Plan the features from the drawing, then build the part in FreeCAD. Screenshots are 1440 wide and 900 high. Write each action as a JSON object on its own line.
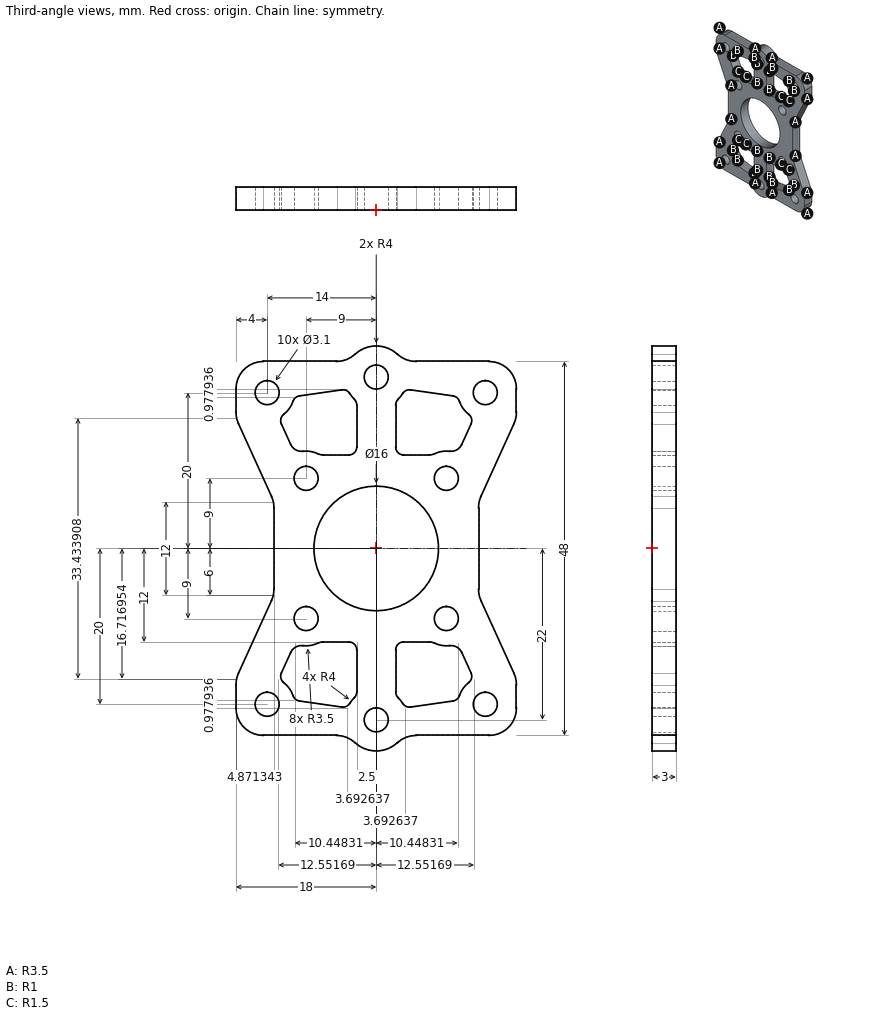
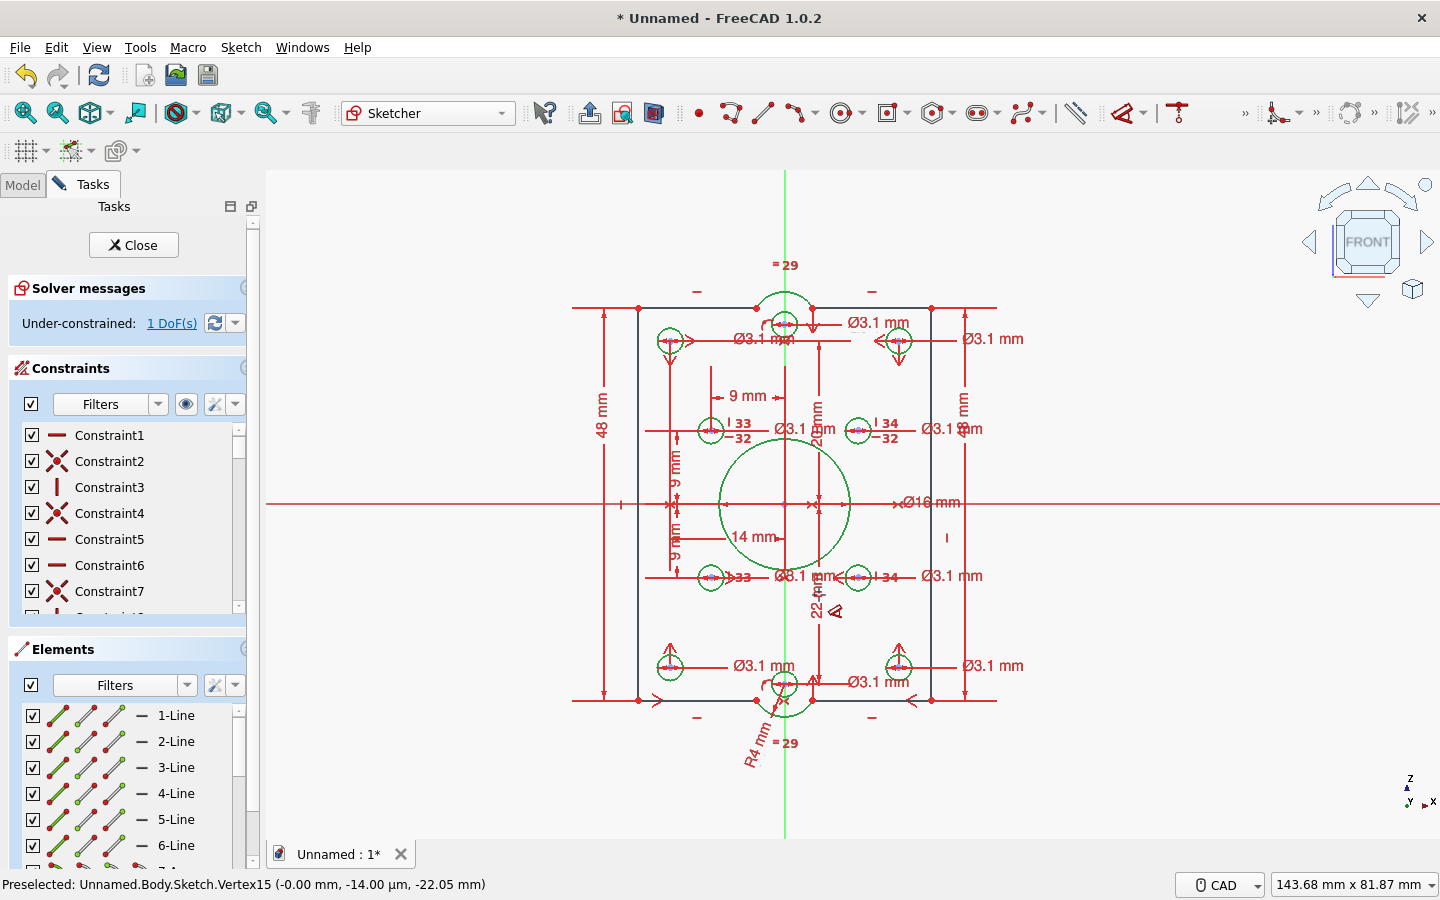
{"action": "left_click", "coordinate": [638, 308]}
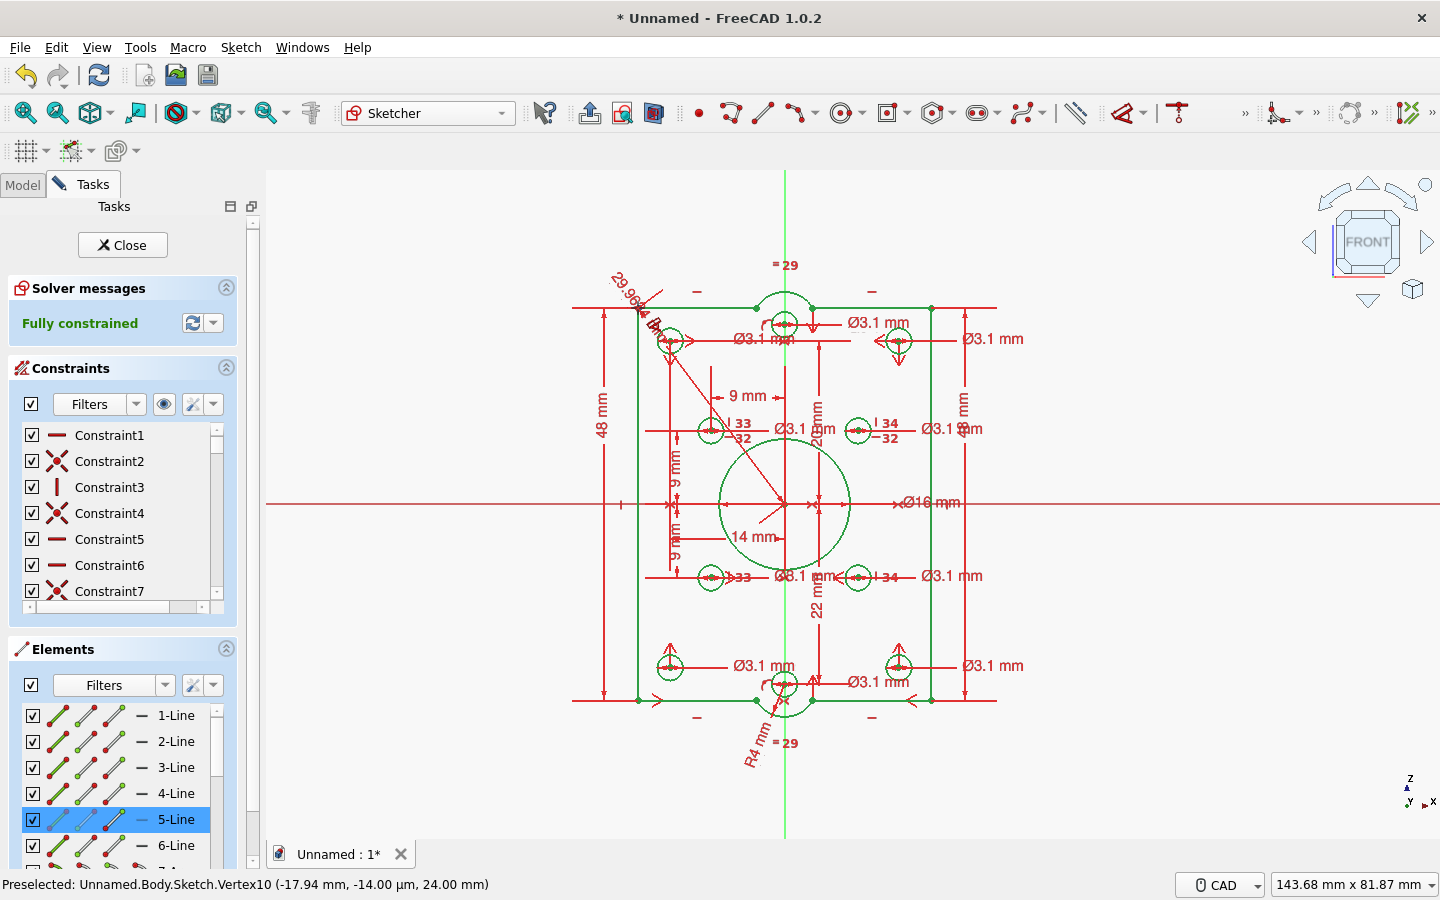
{"action": "left_click", "coordinate": [670, 341]}
{"action": "left_click", "coordinate": [654, 274]}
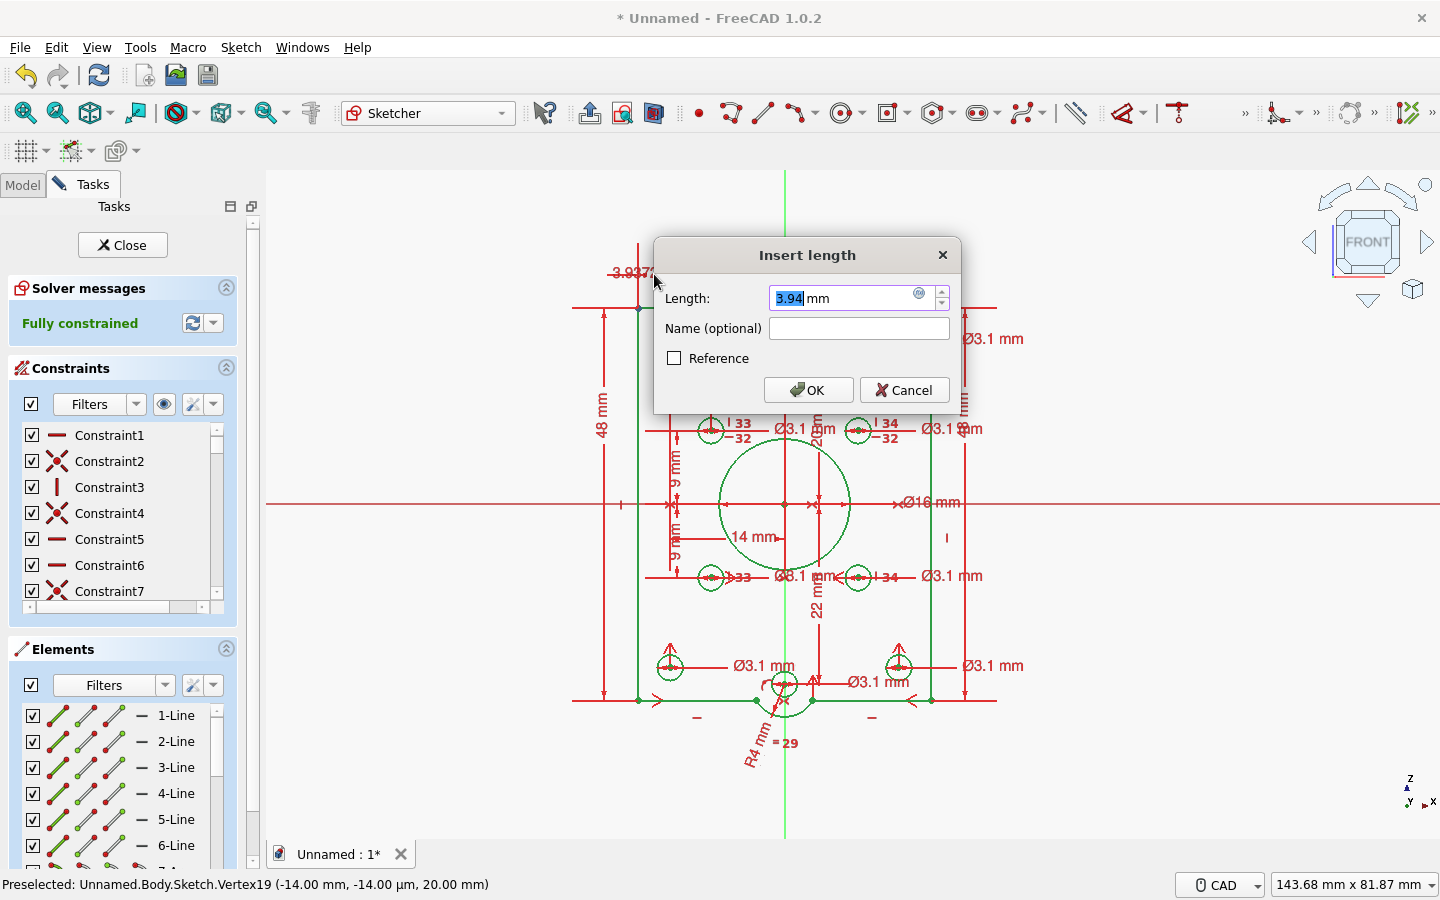
{"action": "type", "text": "4"}
{"action": "key", "text": "Return"}
{"action": "key", "text": "Escape"}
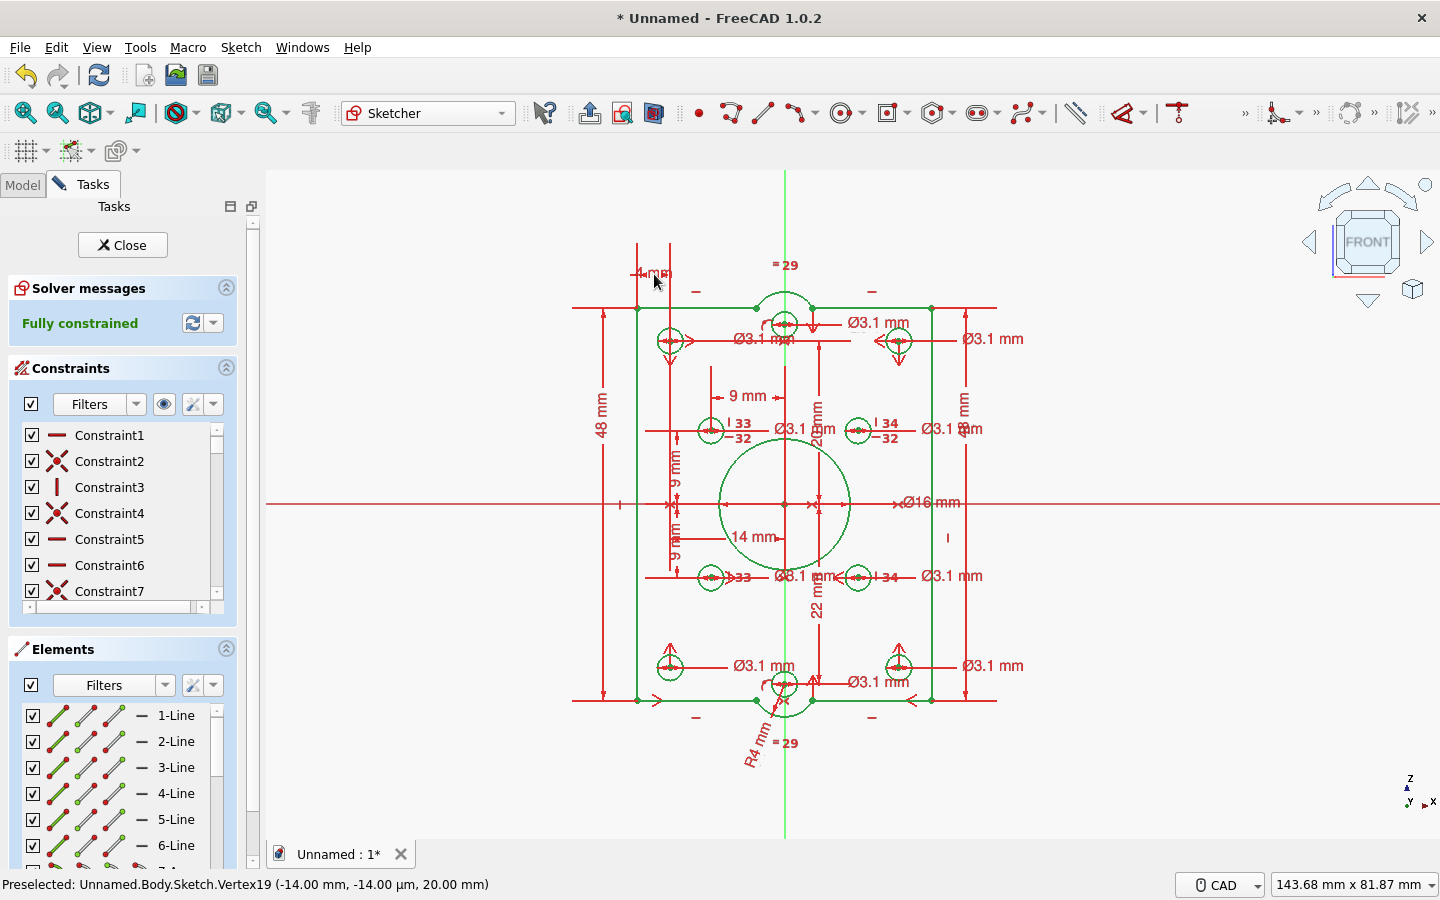
{"action": "left_click", "coordinate": [123, 245]}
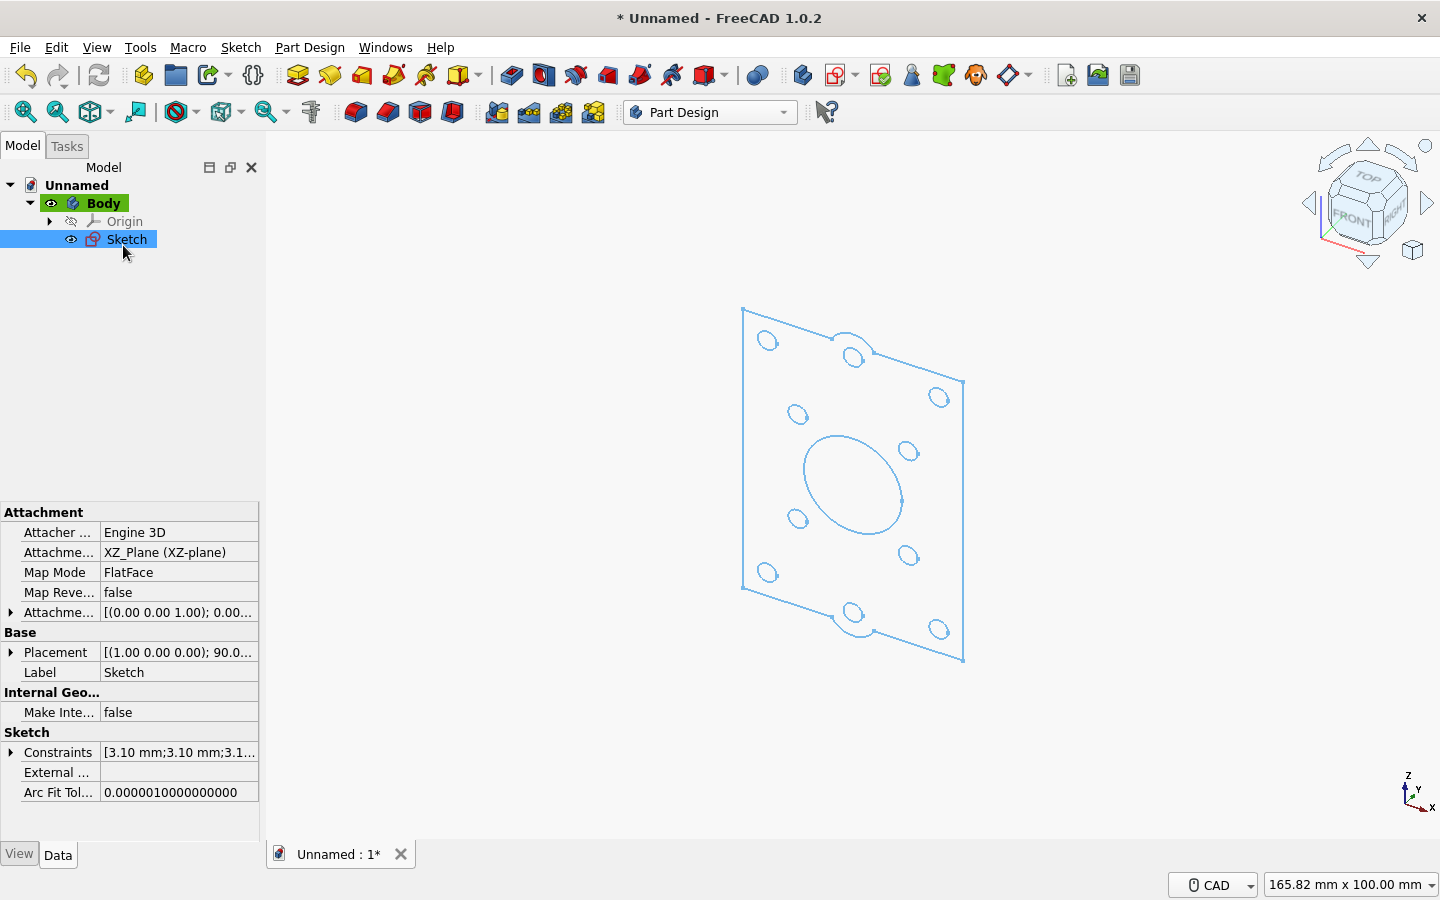
{"action": "left_click", "coordinate": [298, 76]}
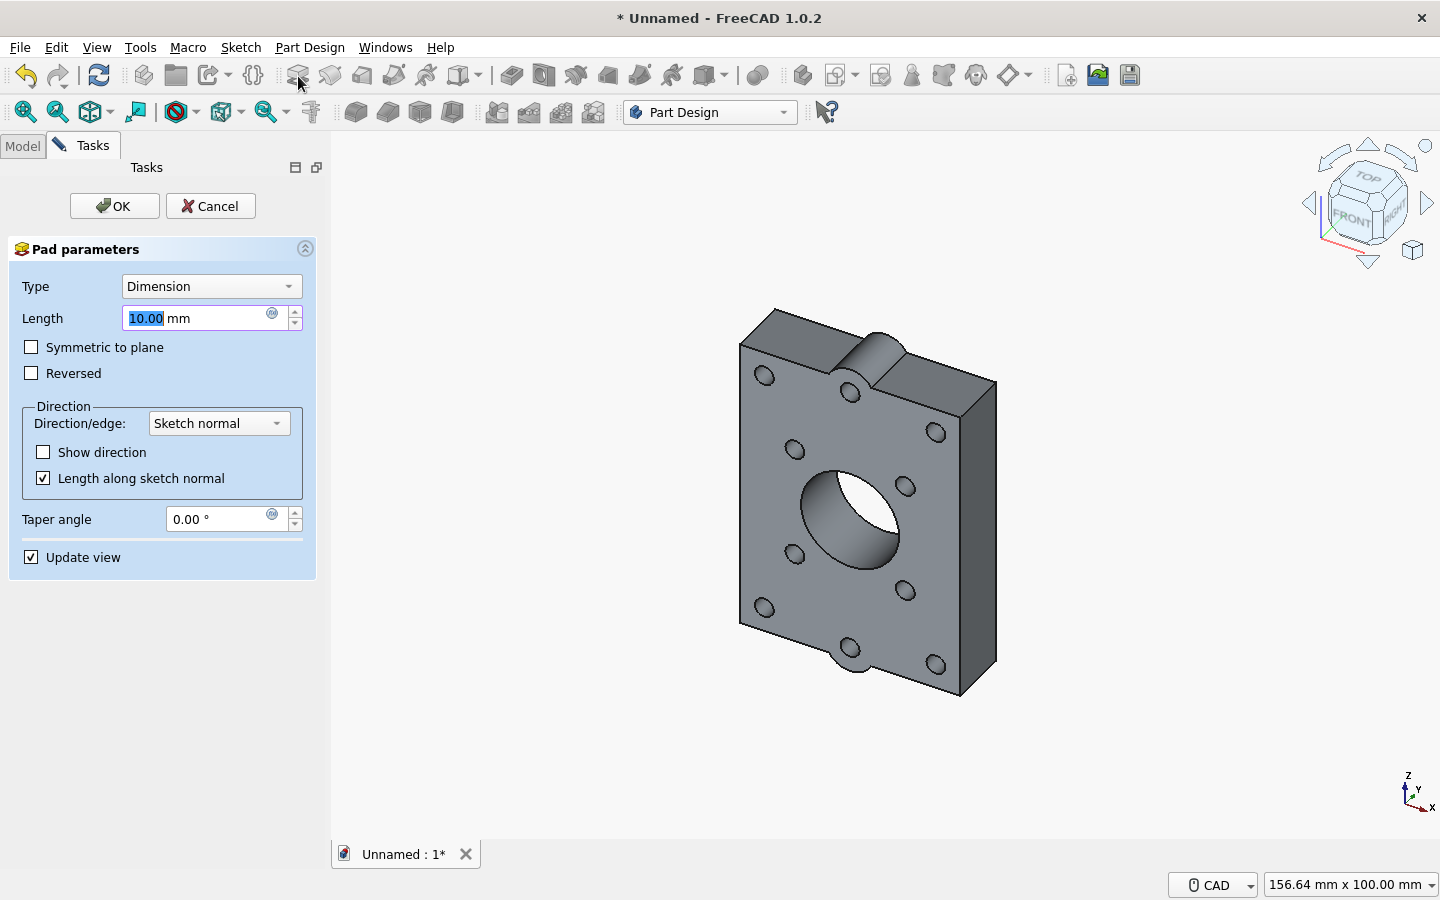
{"action": "type", "text": "3"}
{"action": "key", "text": "Tab"}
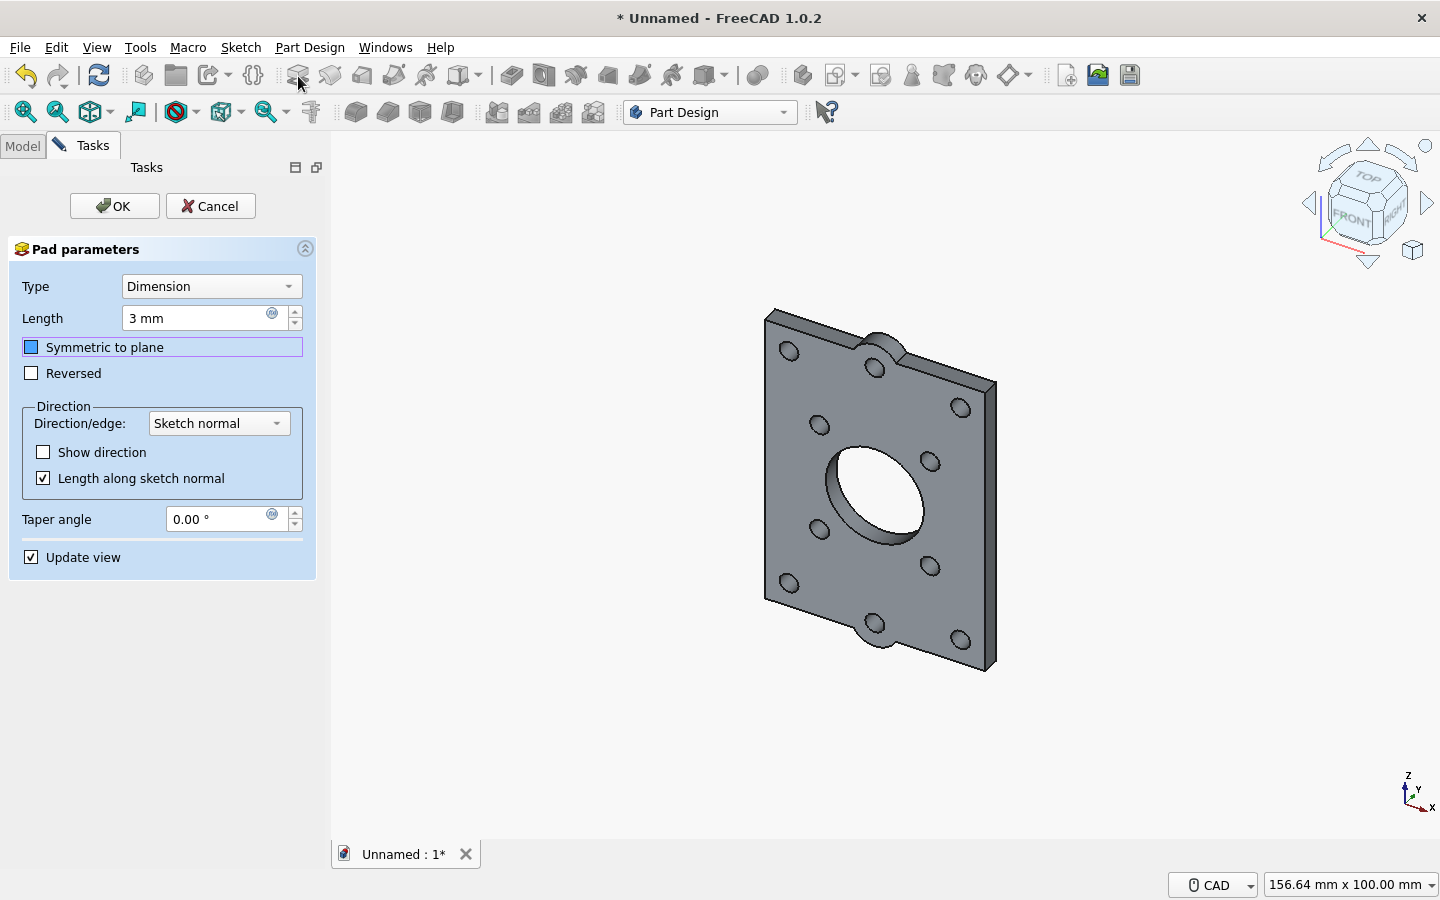
{"action": "left_click", "coordinate": [30, 373]}